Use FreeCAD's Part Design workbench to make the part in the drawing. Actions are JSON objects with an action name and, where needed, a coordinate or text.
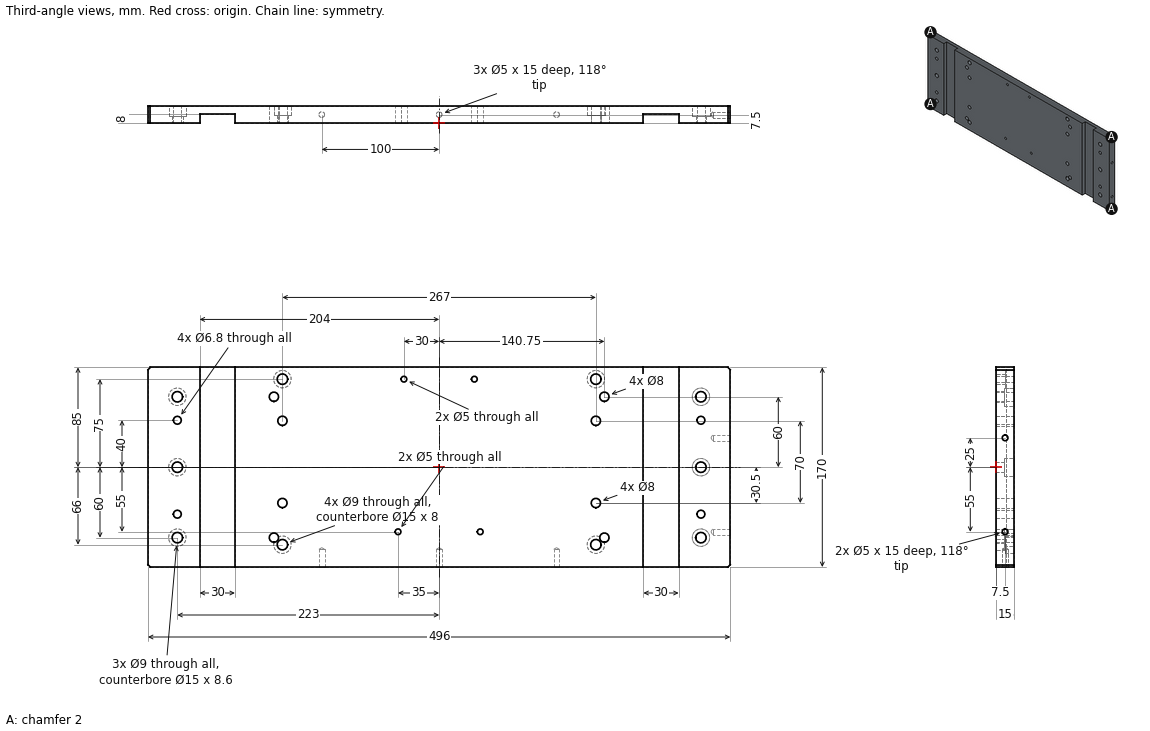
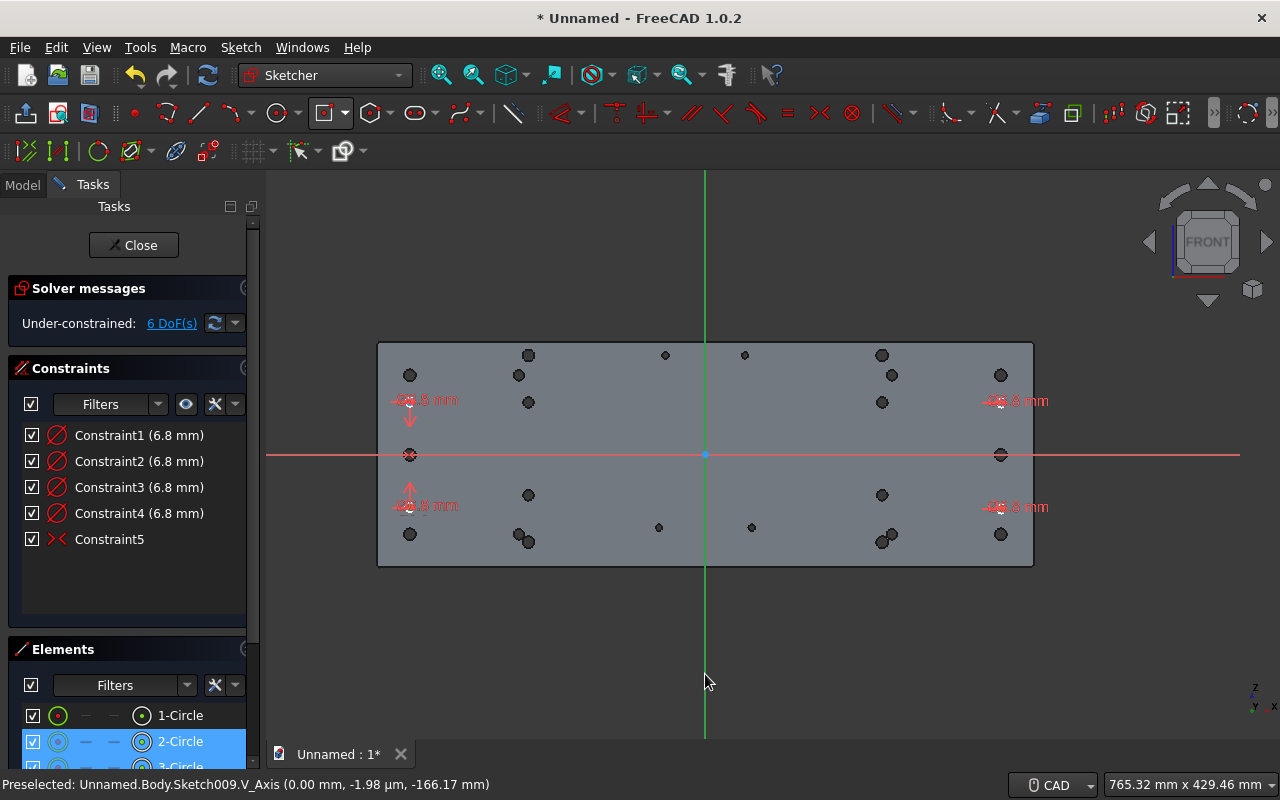
{"action": "left_click", "coordinate": [820, 114]}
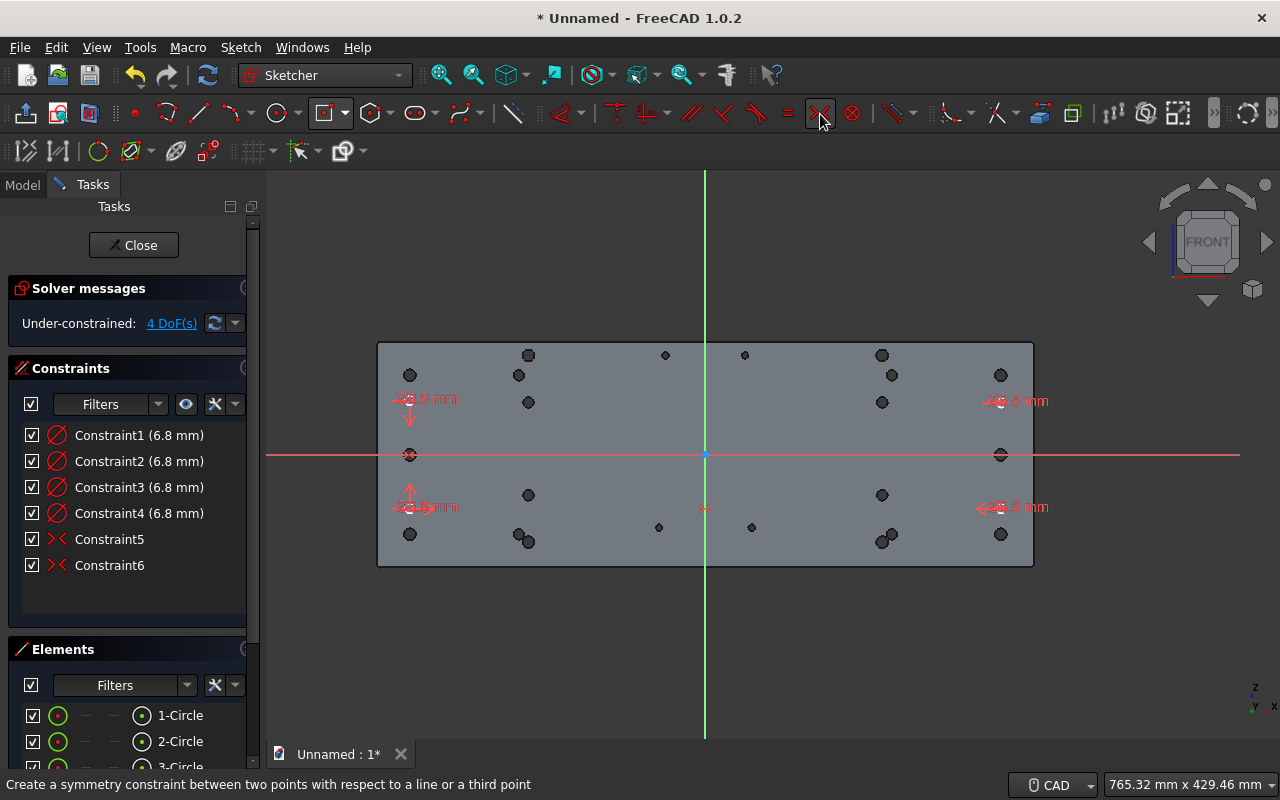
{"action": "left_click", "coordinate": [410, 401]}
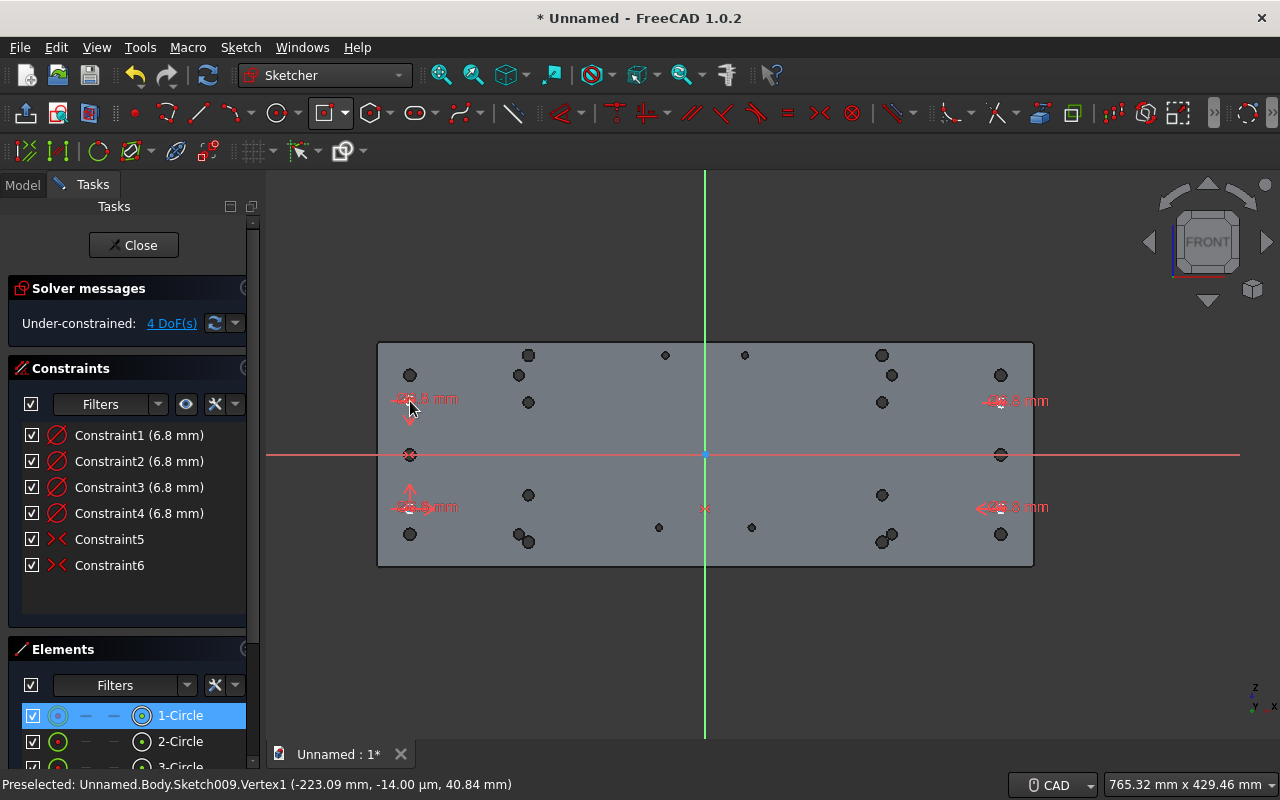
{"action": "left_click", "coordinate": [1001, 403]}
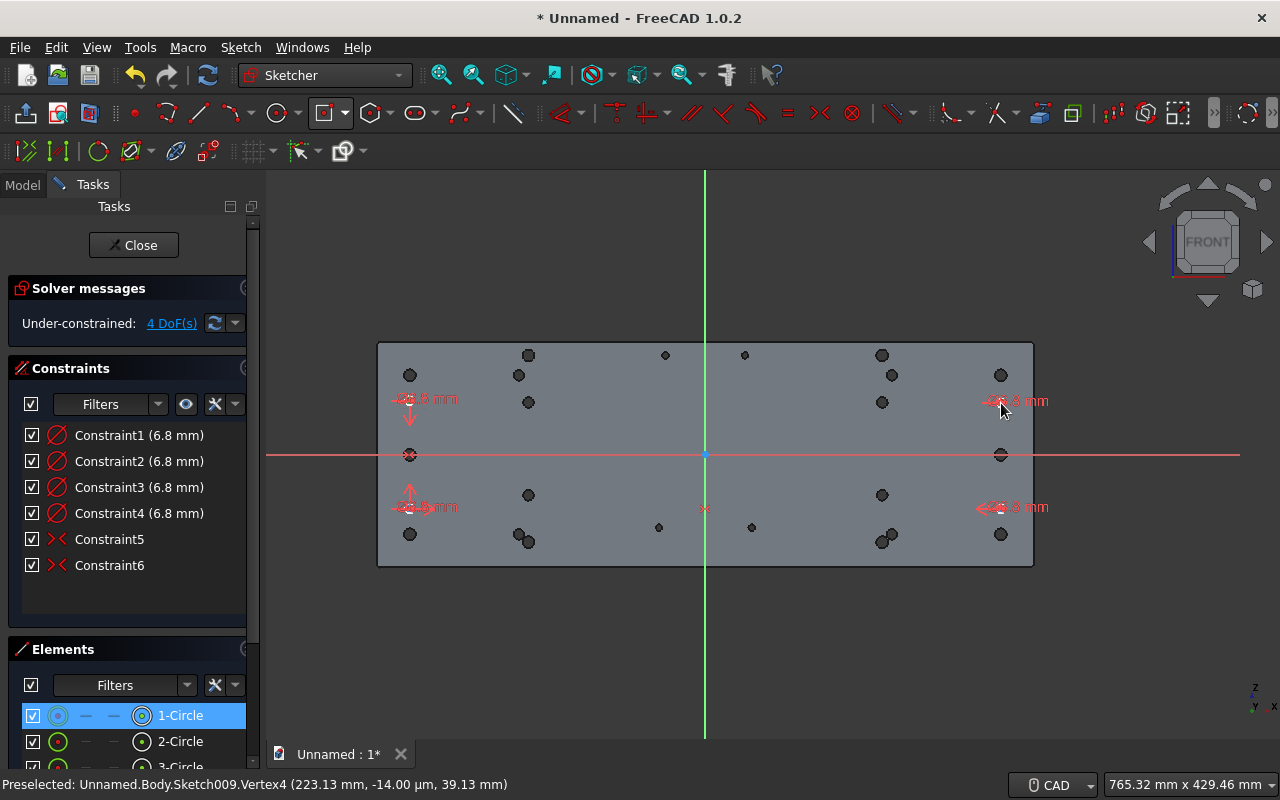
{"action": "left_click", "coordinate": [705, 674]}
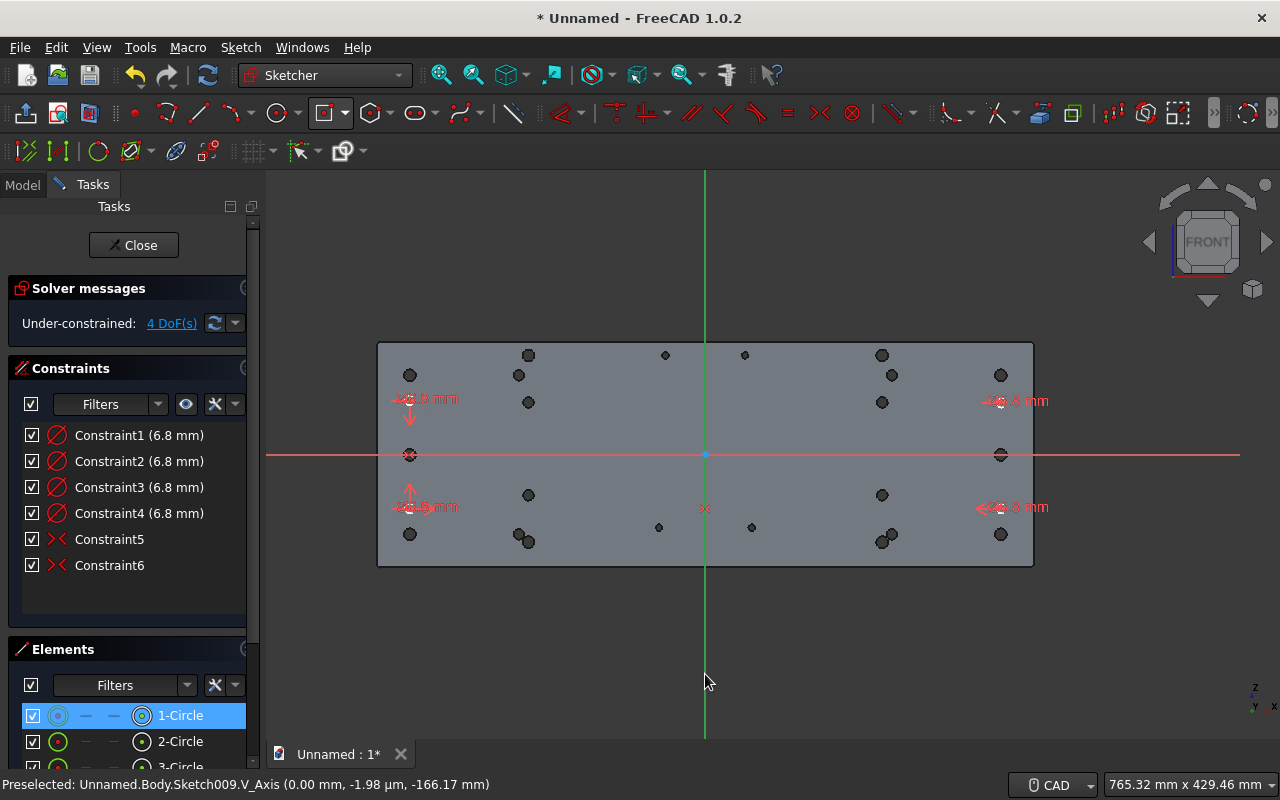
{"action": "left_click", "coordinate": [820, 114]}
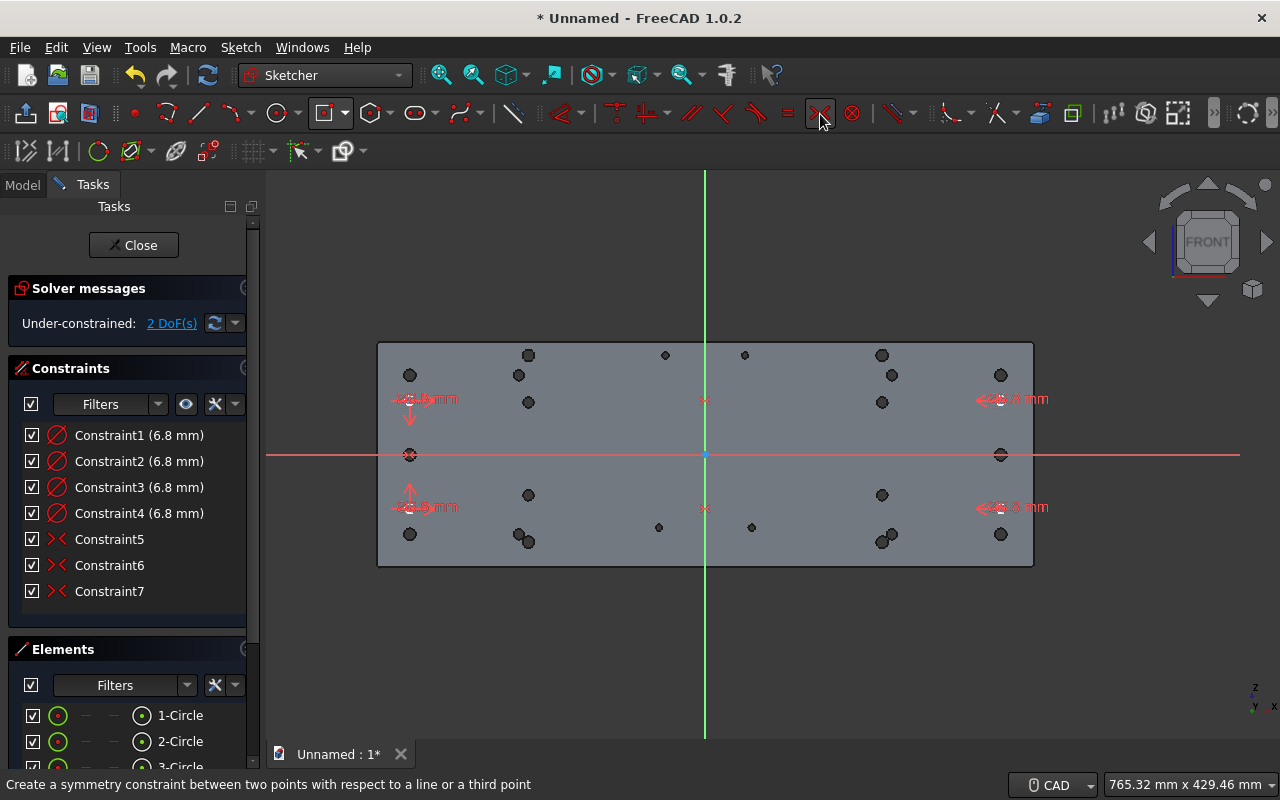
{"action": "left_click", "coordinate": [560, 114]}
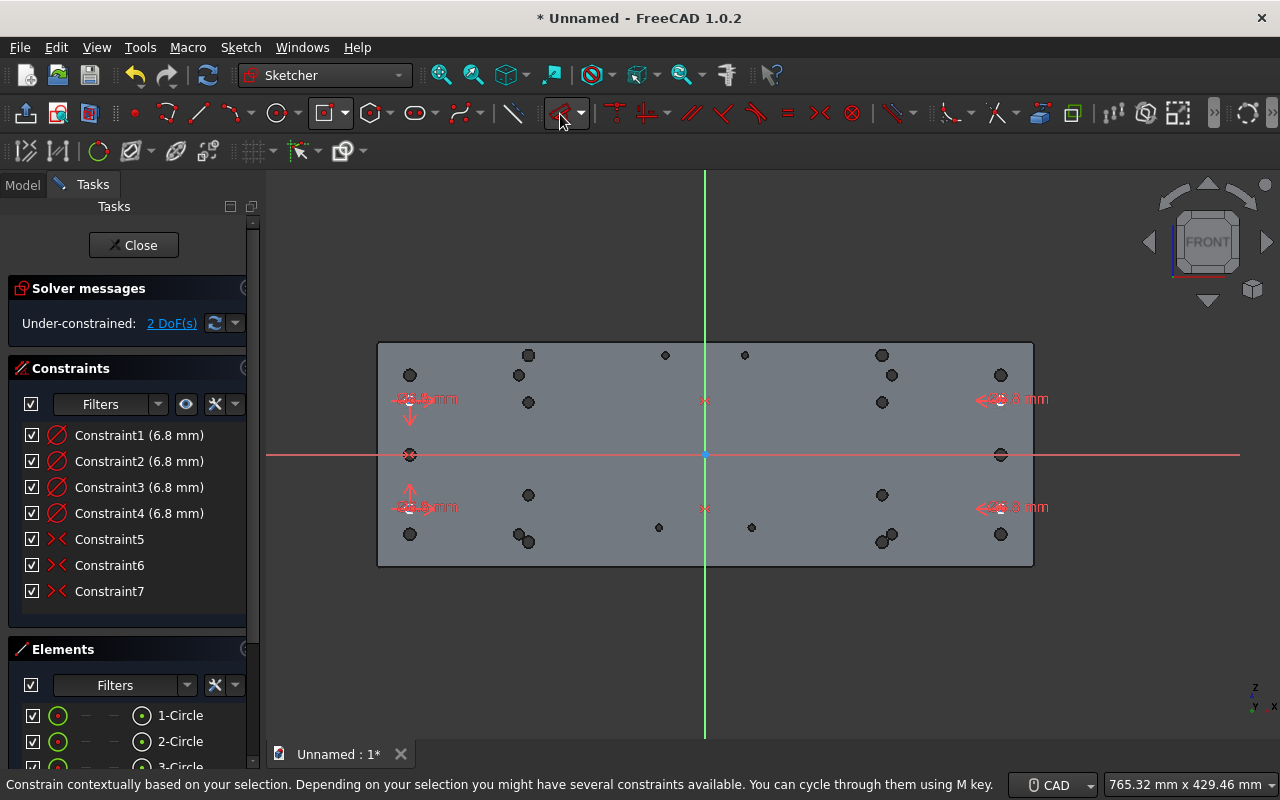
{"action": "left_click", "coordinate": [410, 401]}
{"action": "left_click", "coordinate": [376, 428]}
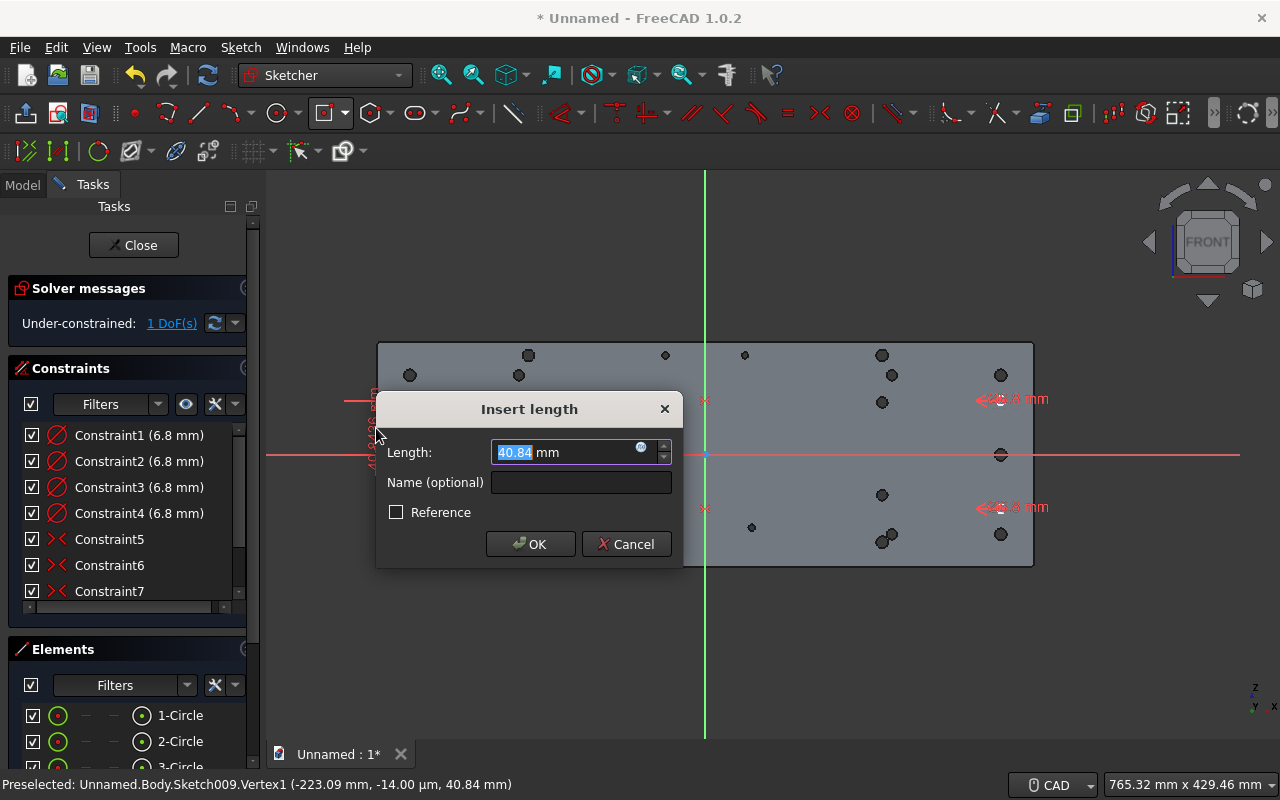
{"action": "type", "text": "40"}
{"action": "key", "text": "Return"}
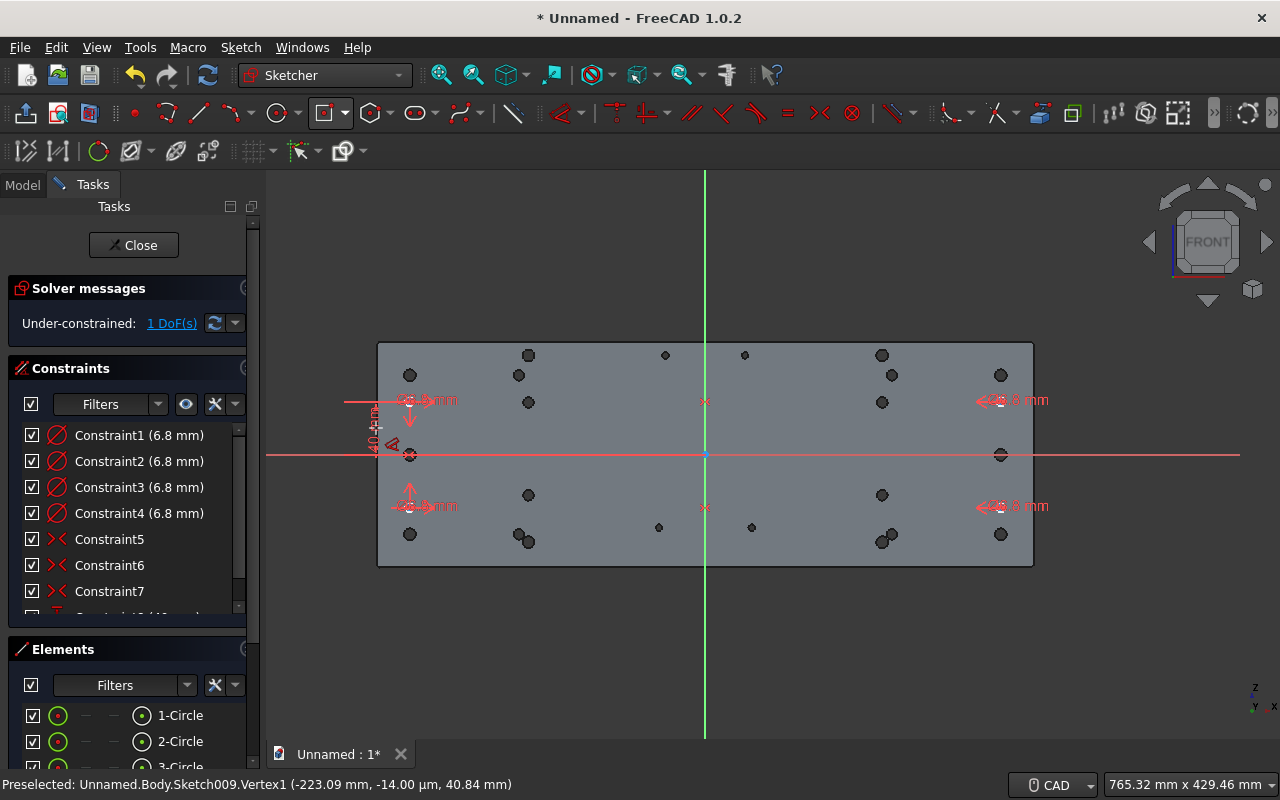
{"action": "left_click", "coordinate": [410, 402]}
{"action": "left_click", "coordinate": [558, 368]}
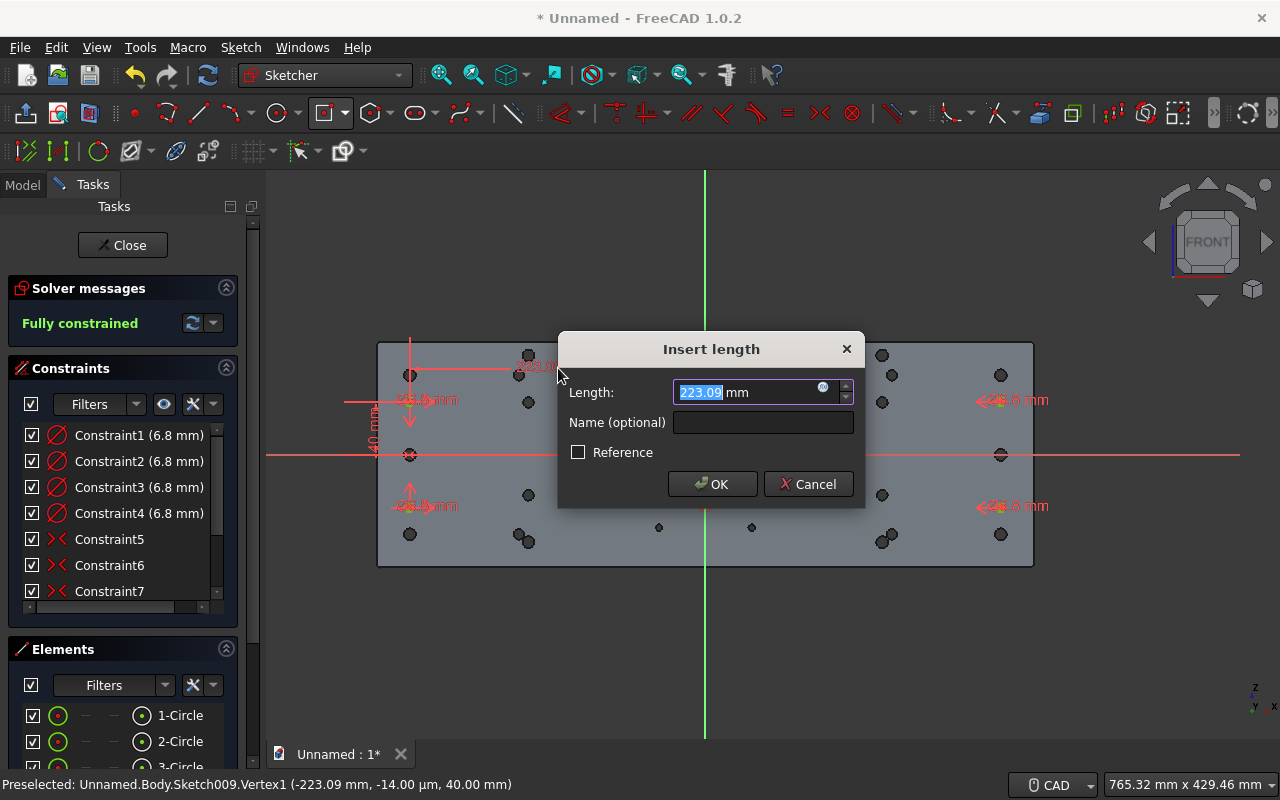
{"action": "type", "text": "223"}
{"action": "key", "text": "Return"}
{"action": "key", "text": "Escape"}